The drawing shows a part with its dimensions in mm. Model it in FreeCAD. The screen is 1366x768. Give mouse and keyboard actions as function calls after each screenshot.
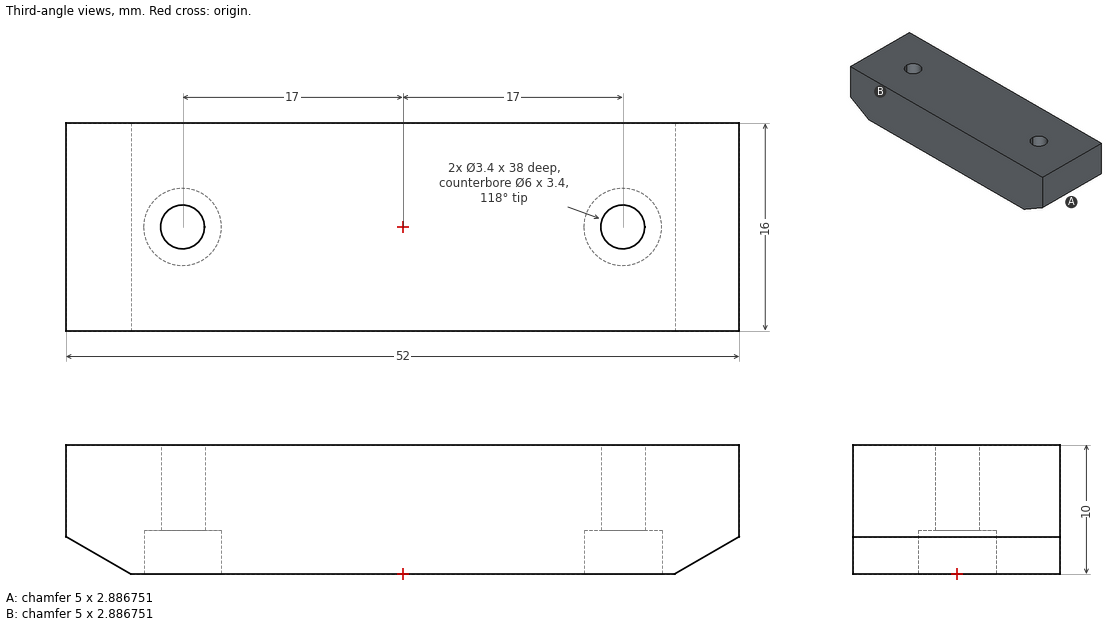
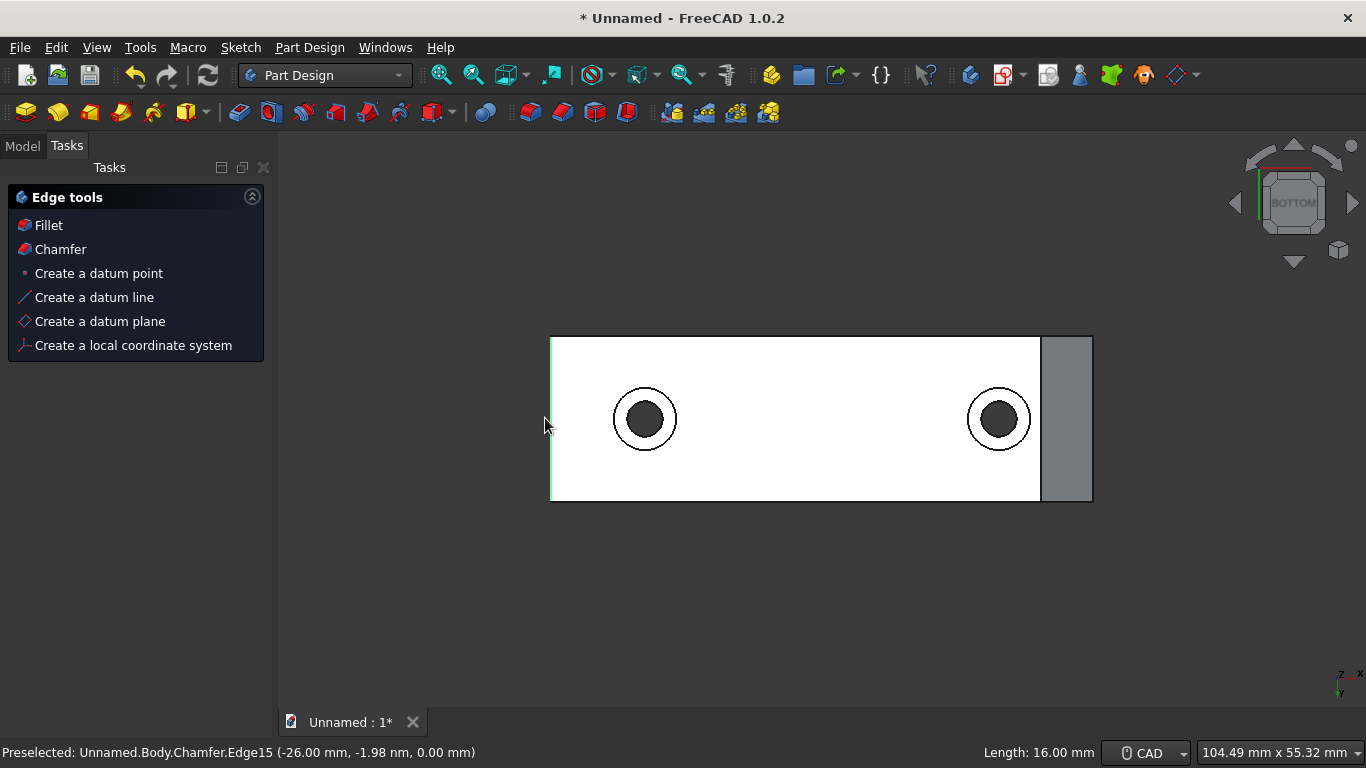
click(564, 112)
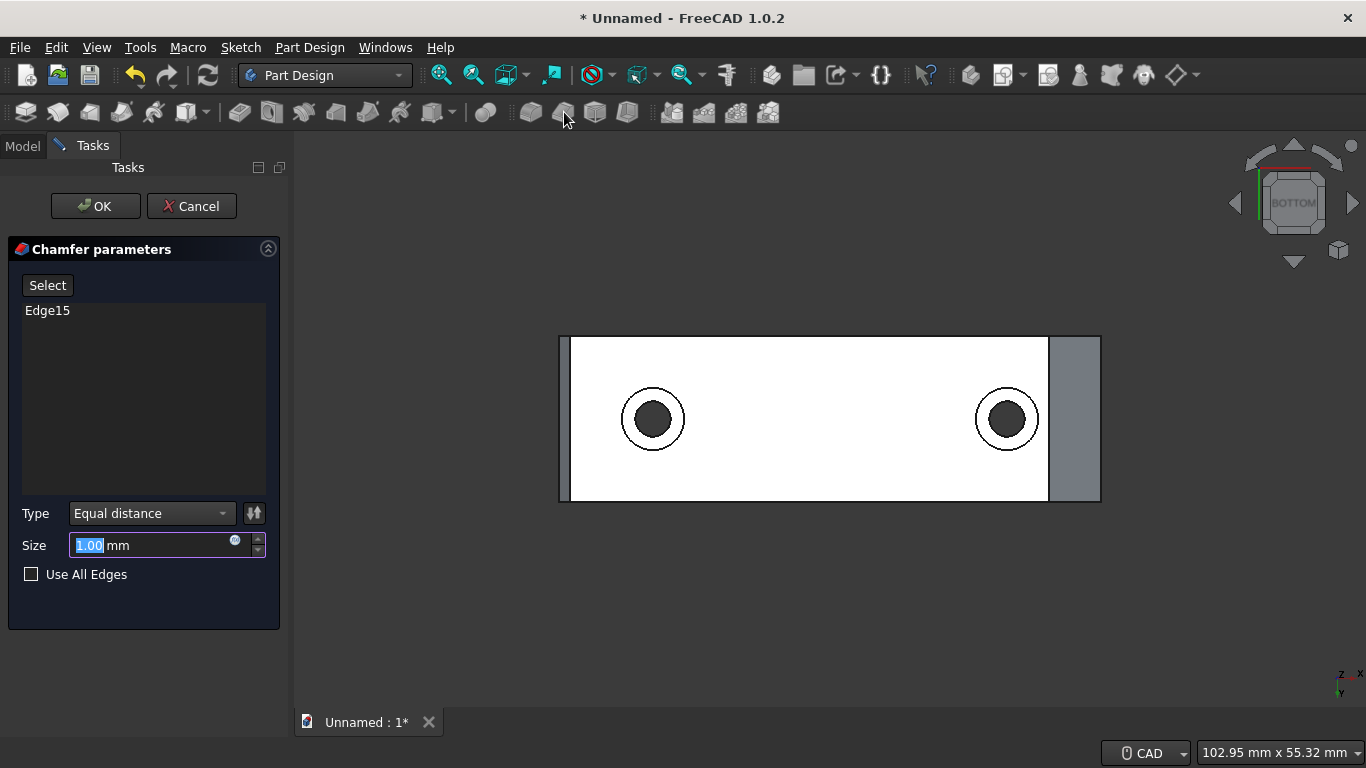
text(5)
key(Tab)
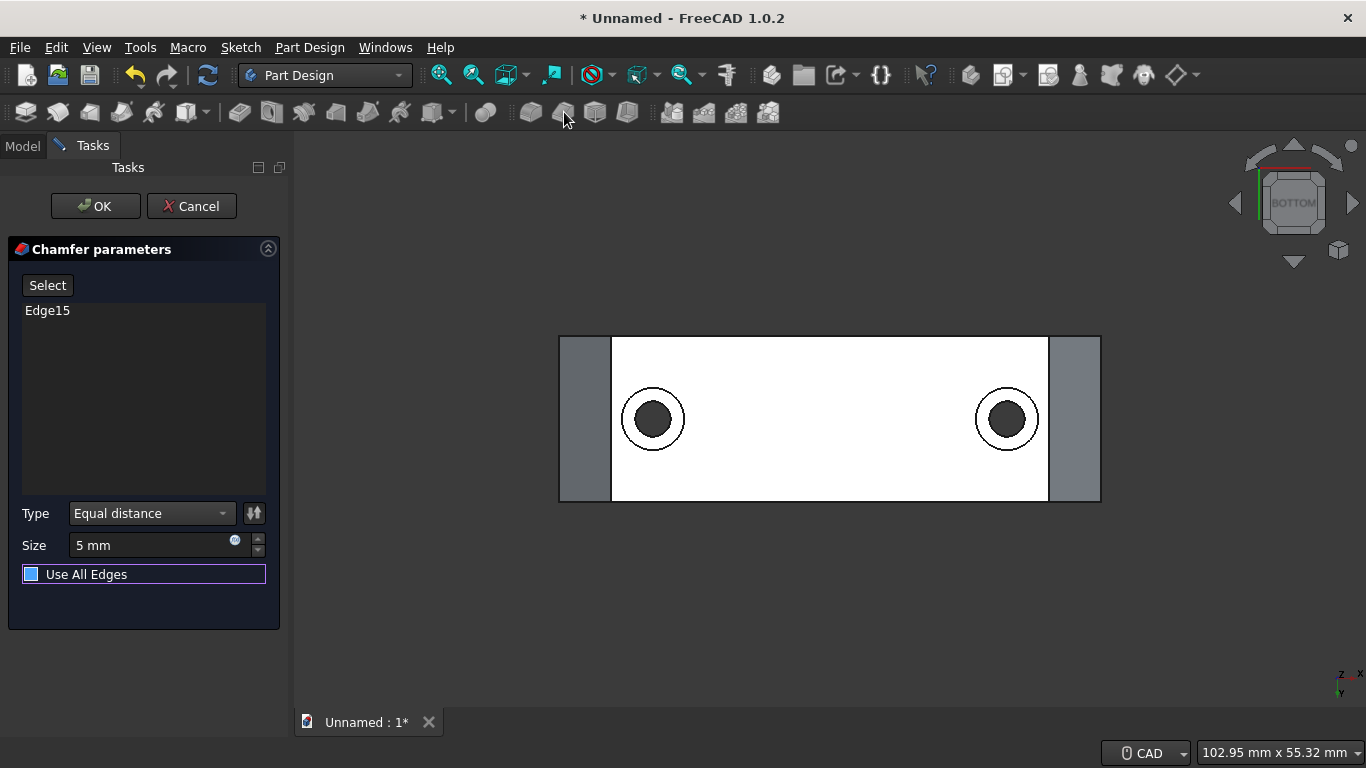
click(153, 514)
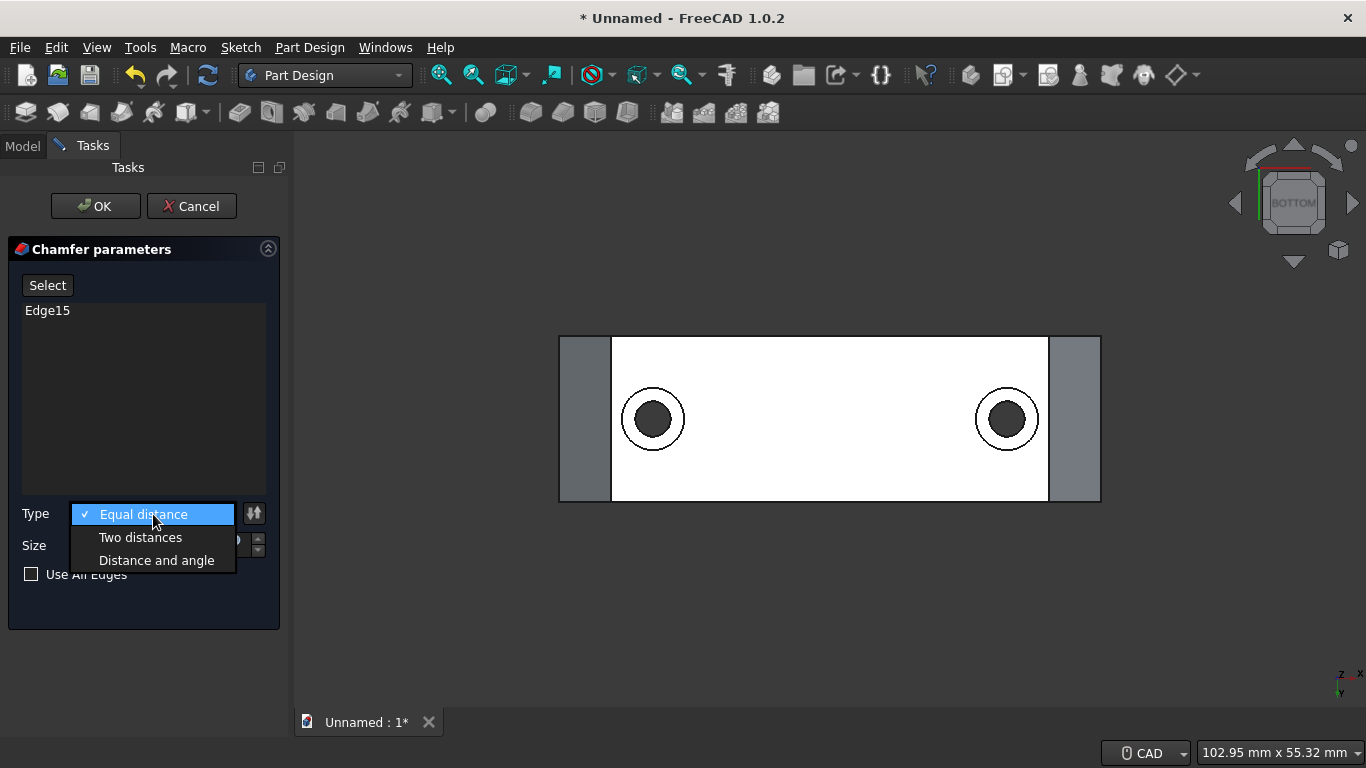
click(152, 538)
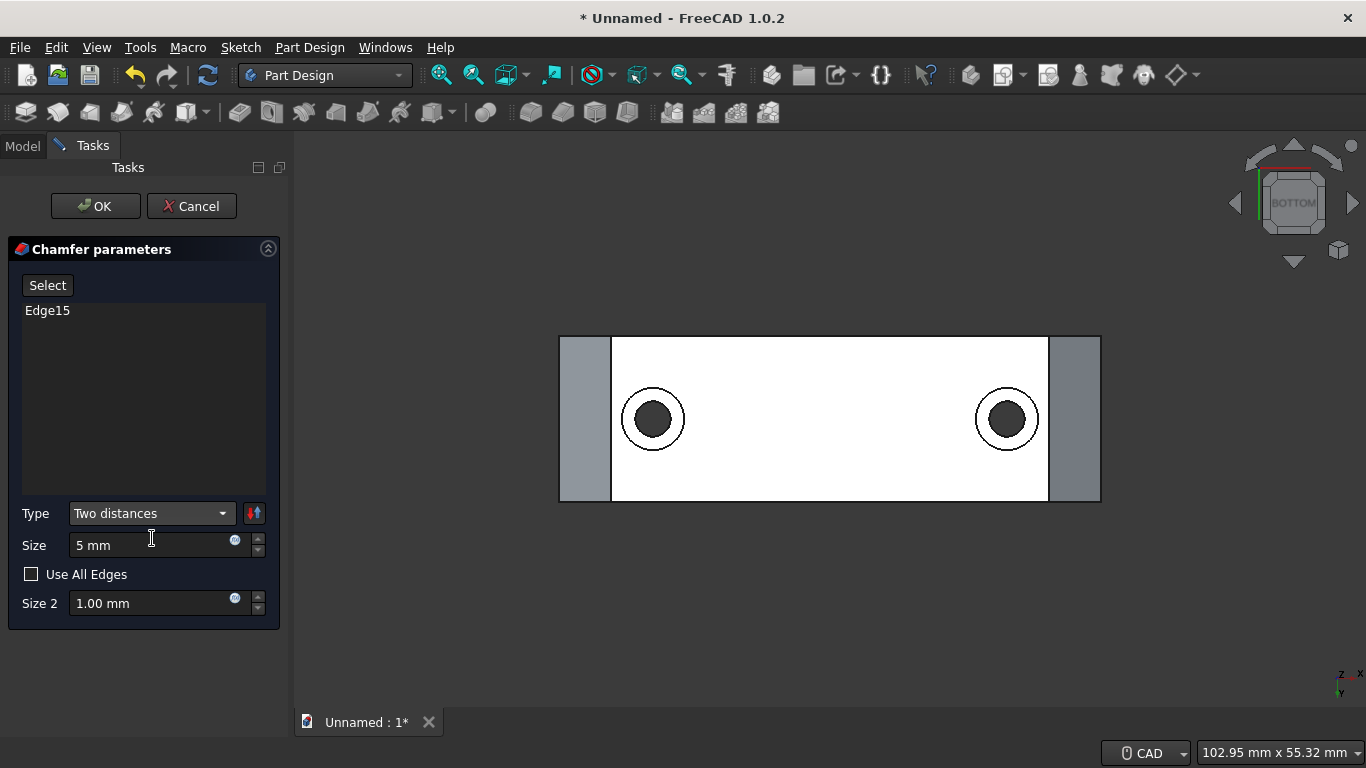
triple_click(160, 603)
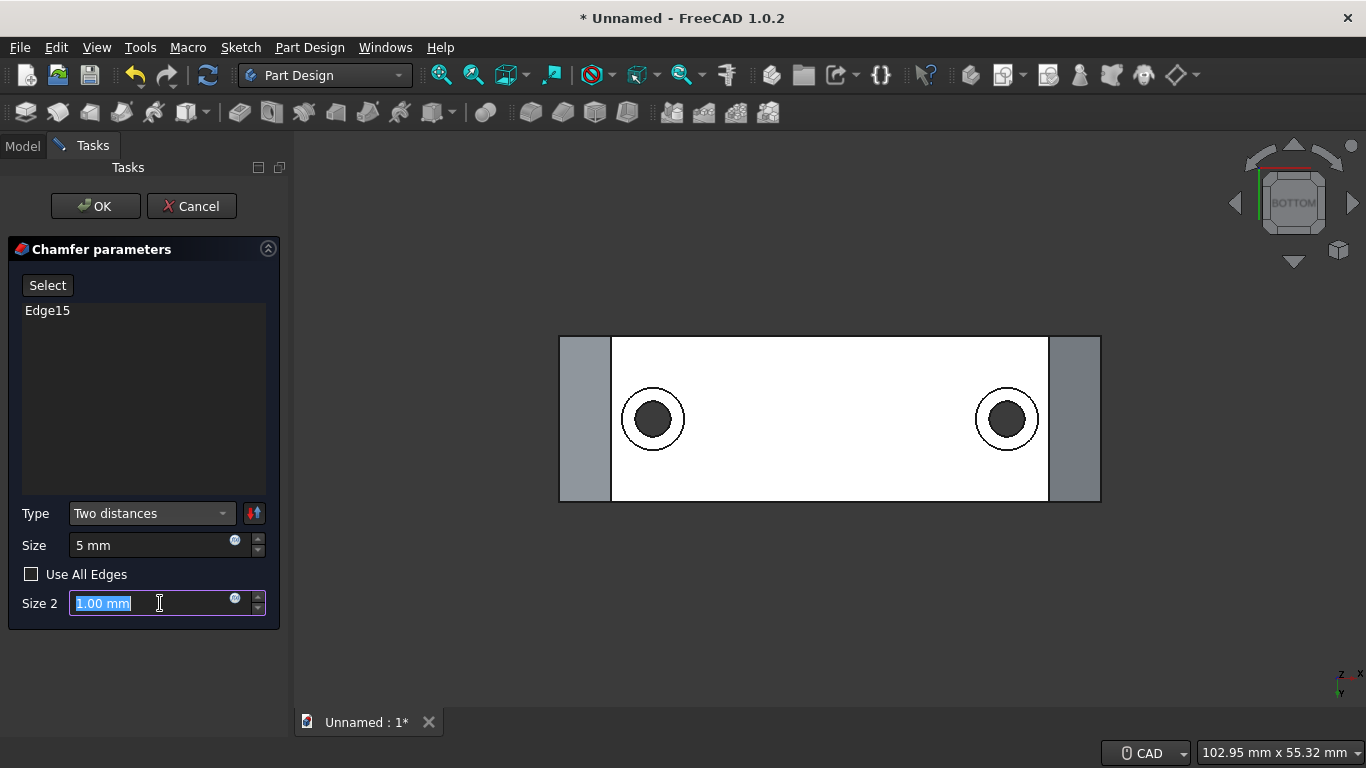
text(2.886751)
key(Tab)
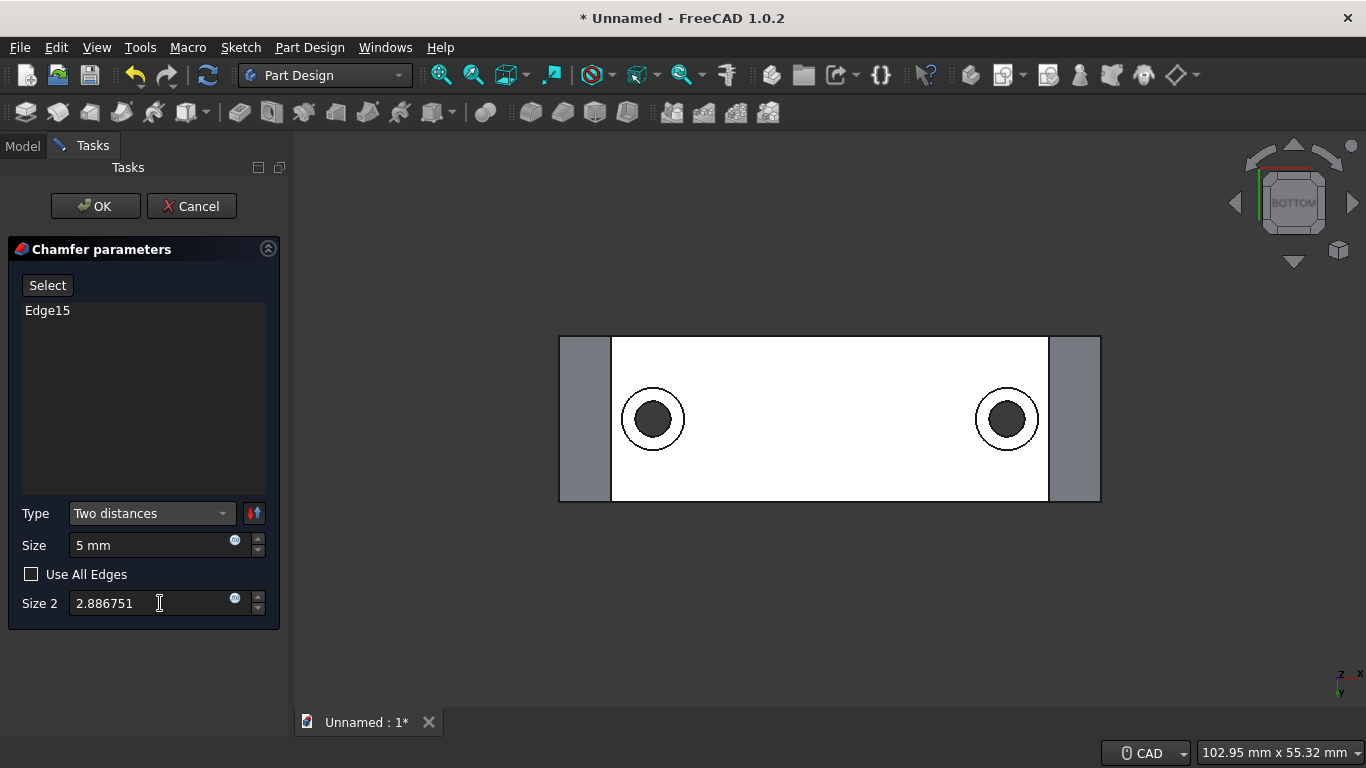
click(96, 206)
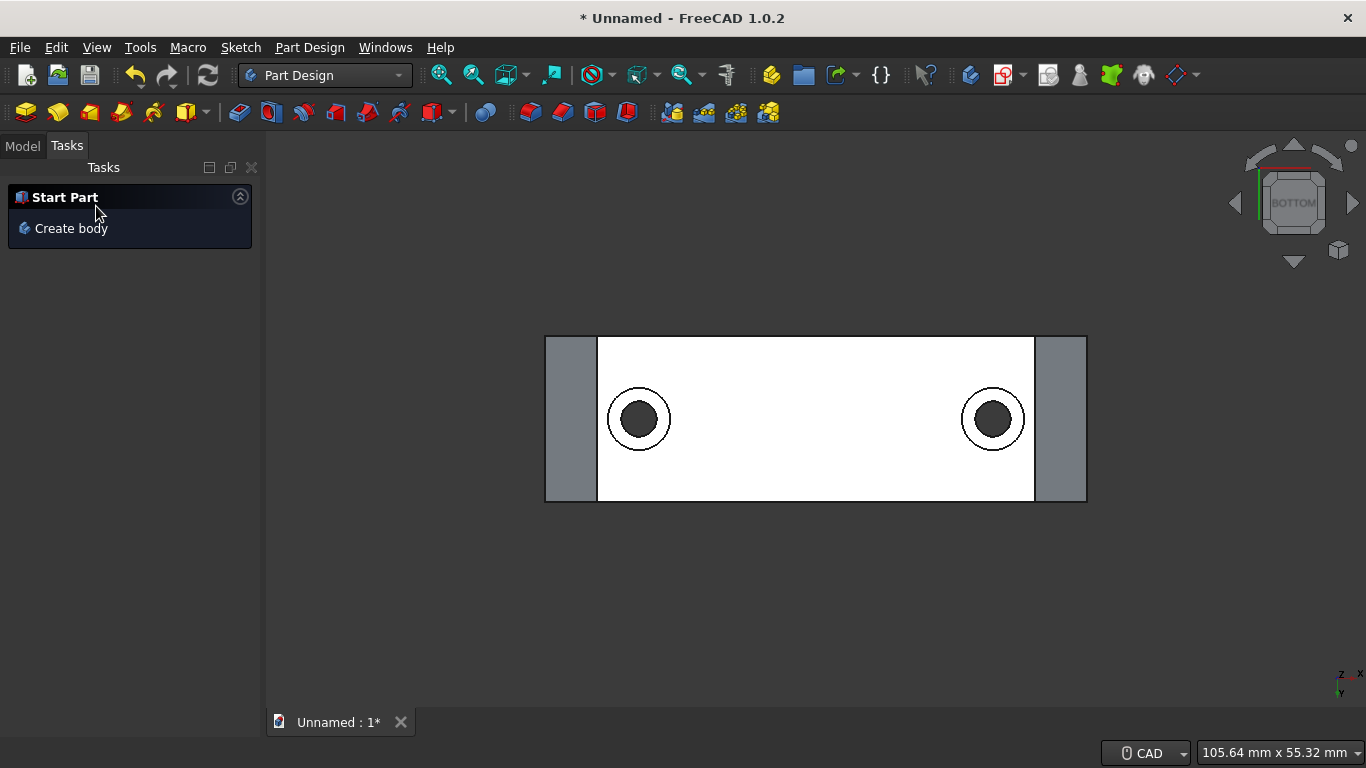
key(0)